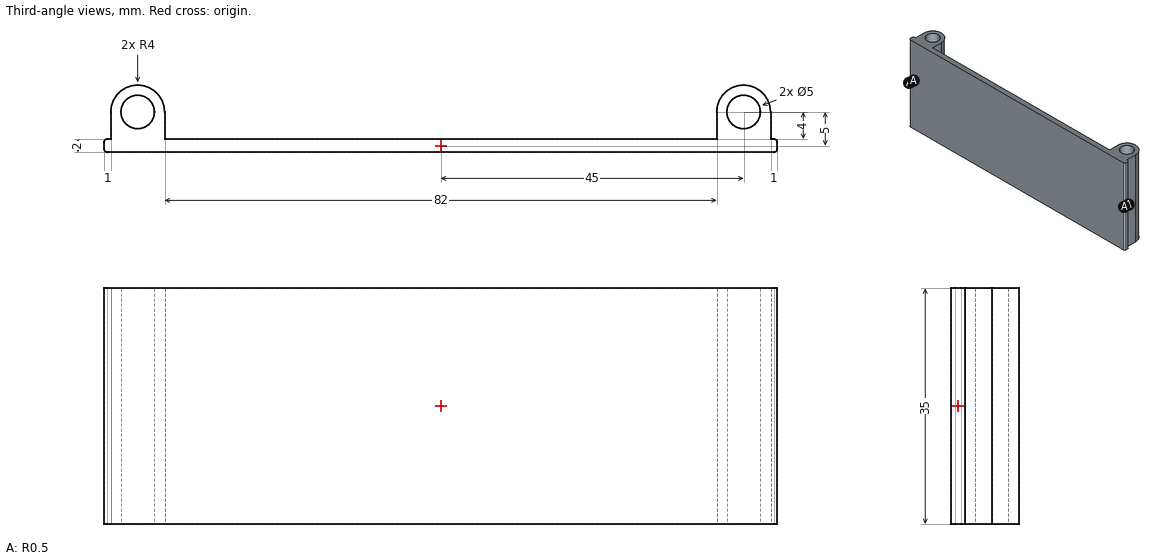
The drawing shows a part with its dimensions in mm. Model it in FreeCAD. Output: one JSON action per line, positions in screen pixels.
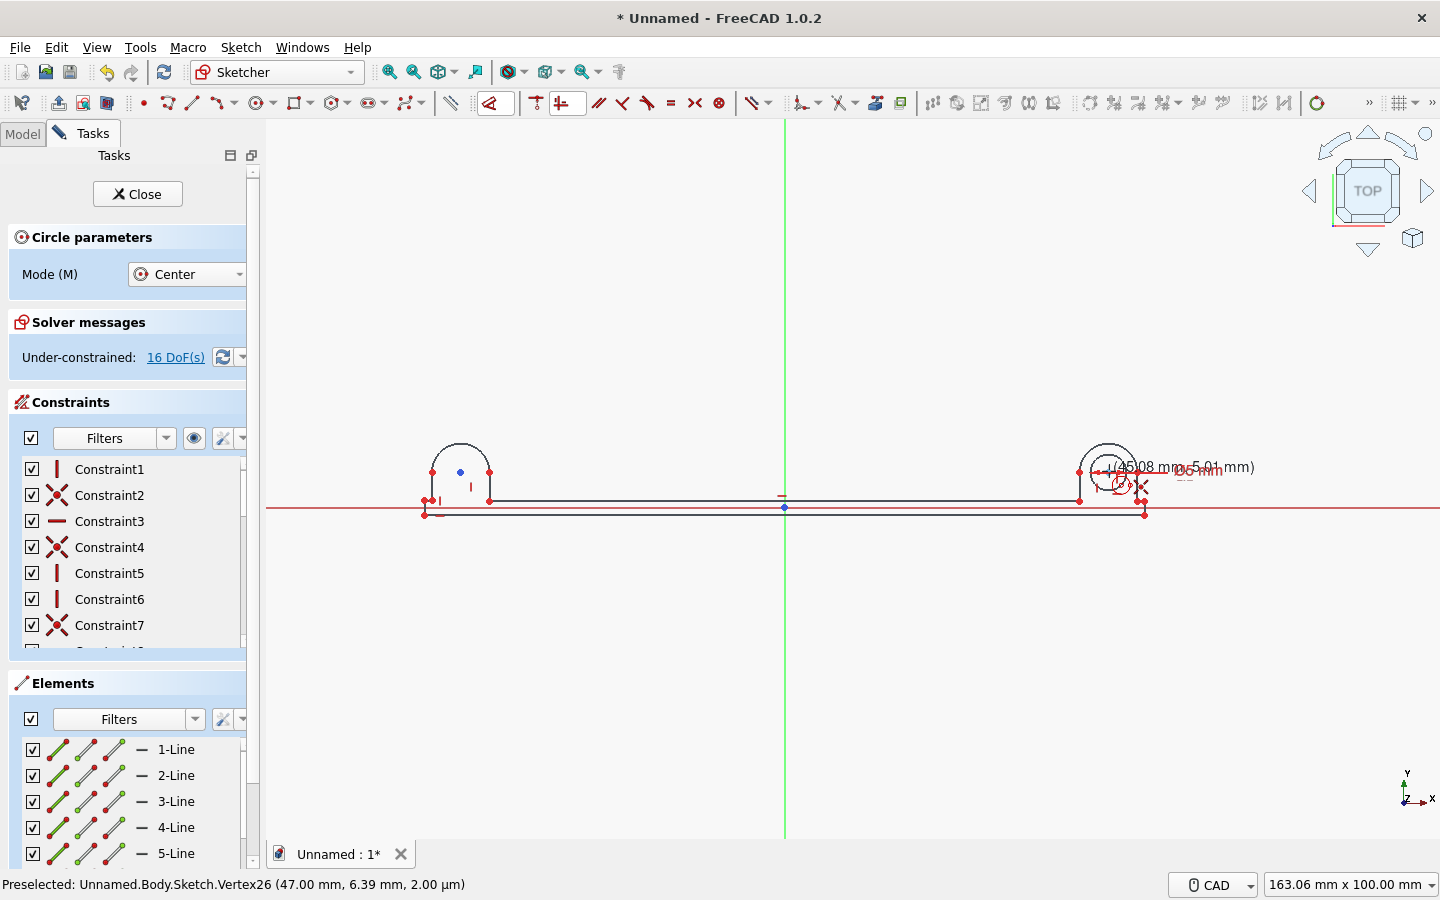
{"action": "scroll", "coordinate": [461, 472], "scroll_direction": "up", "scroll_amount": 2}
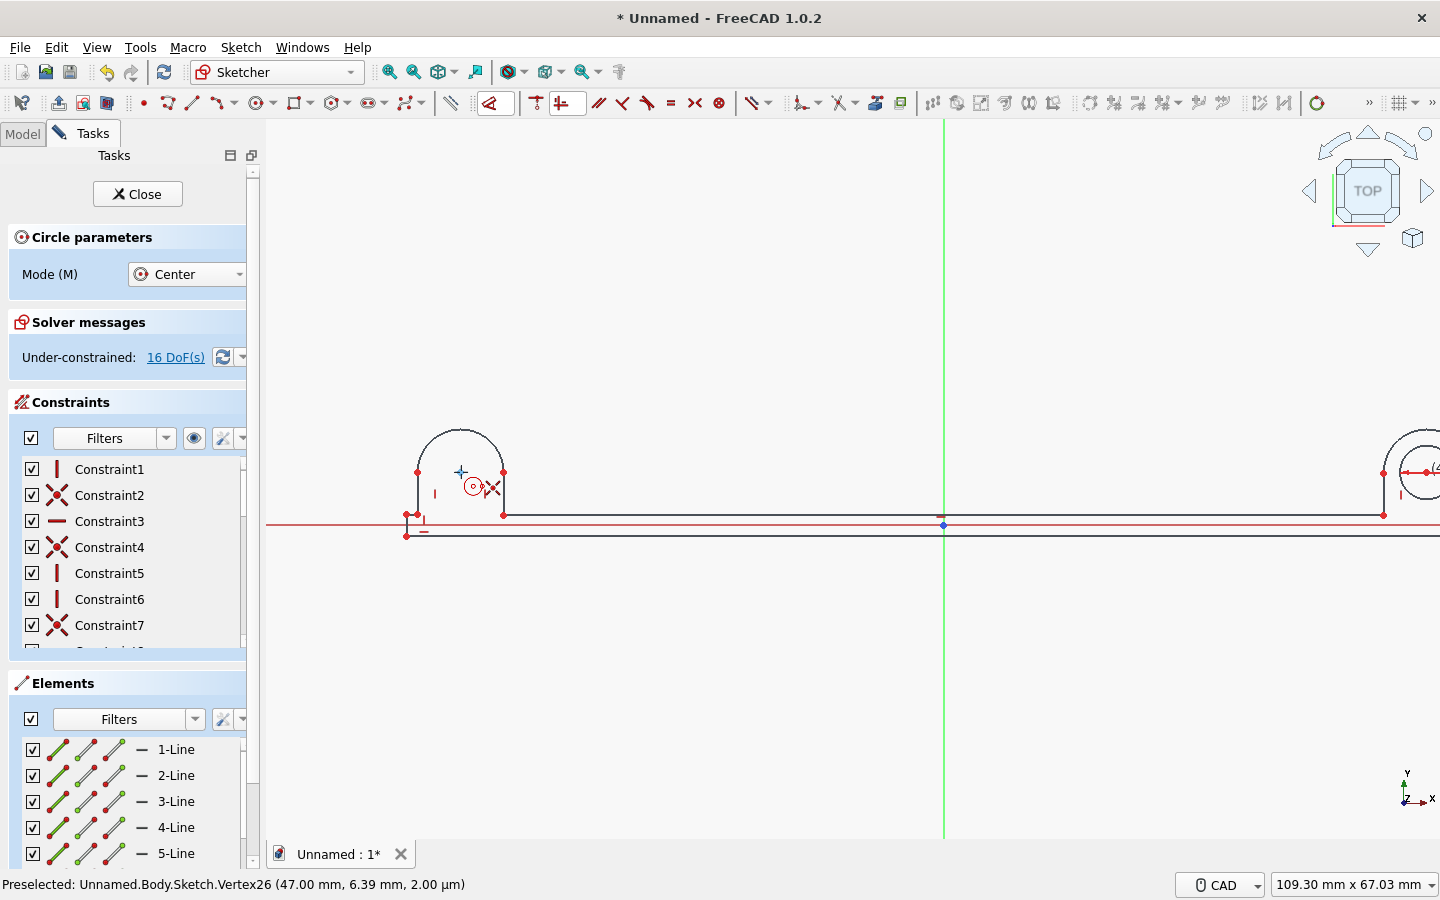
{"action": "left_click", "coordinate": [460, 472]}
{"action": "mouse_move", "coordinate": [479, 453]}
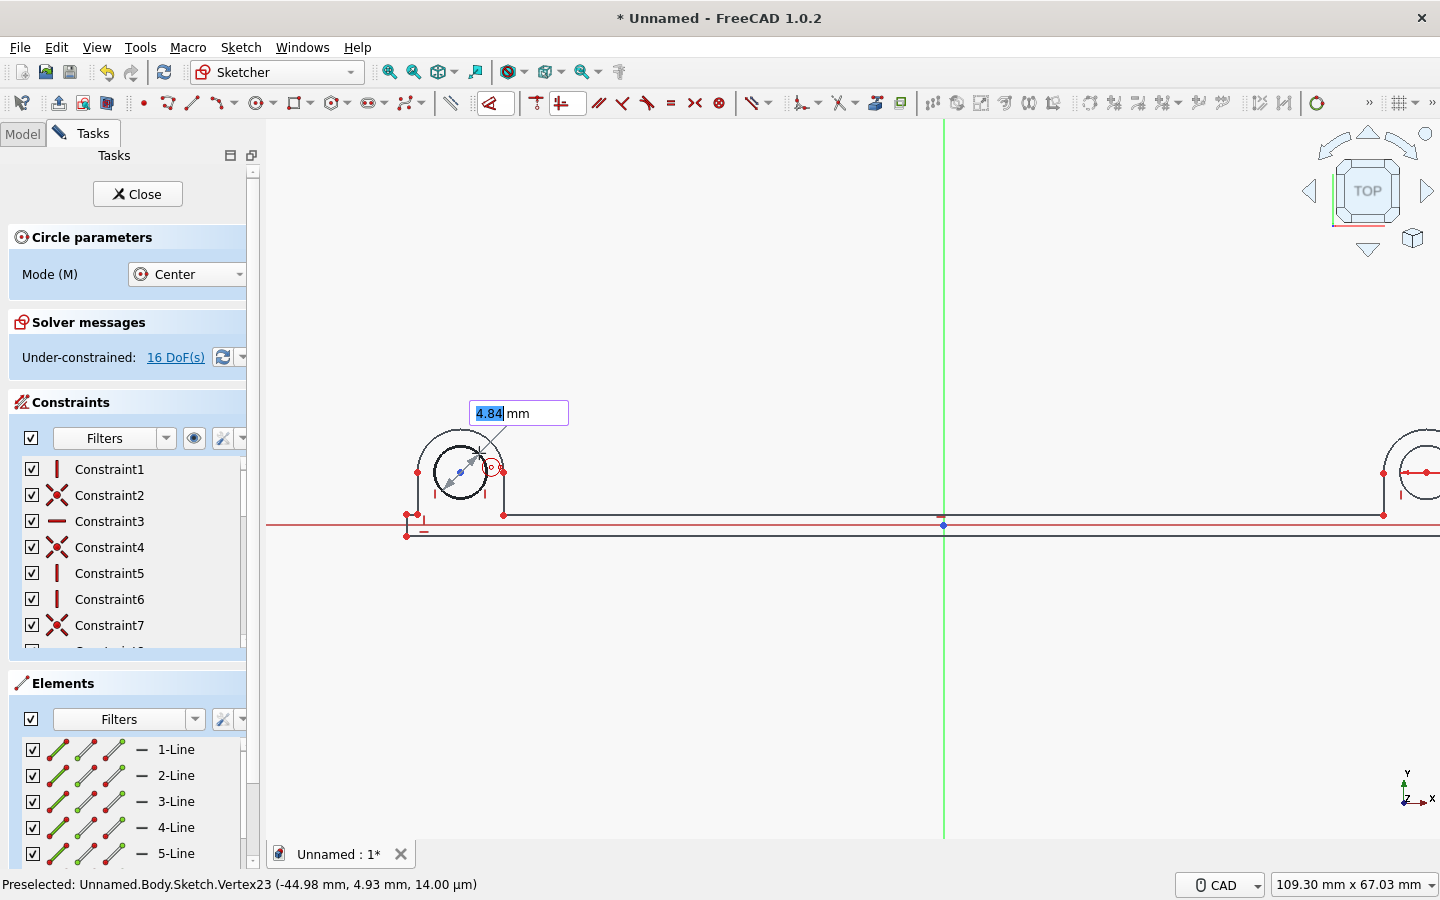
{"action": "type", "text": "5"}
{"action": "key", "text": "Return"}
{"action": "key", "text": "Escape"}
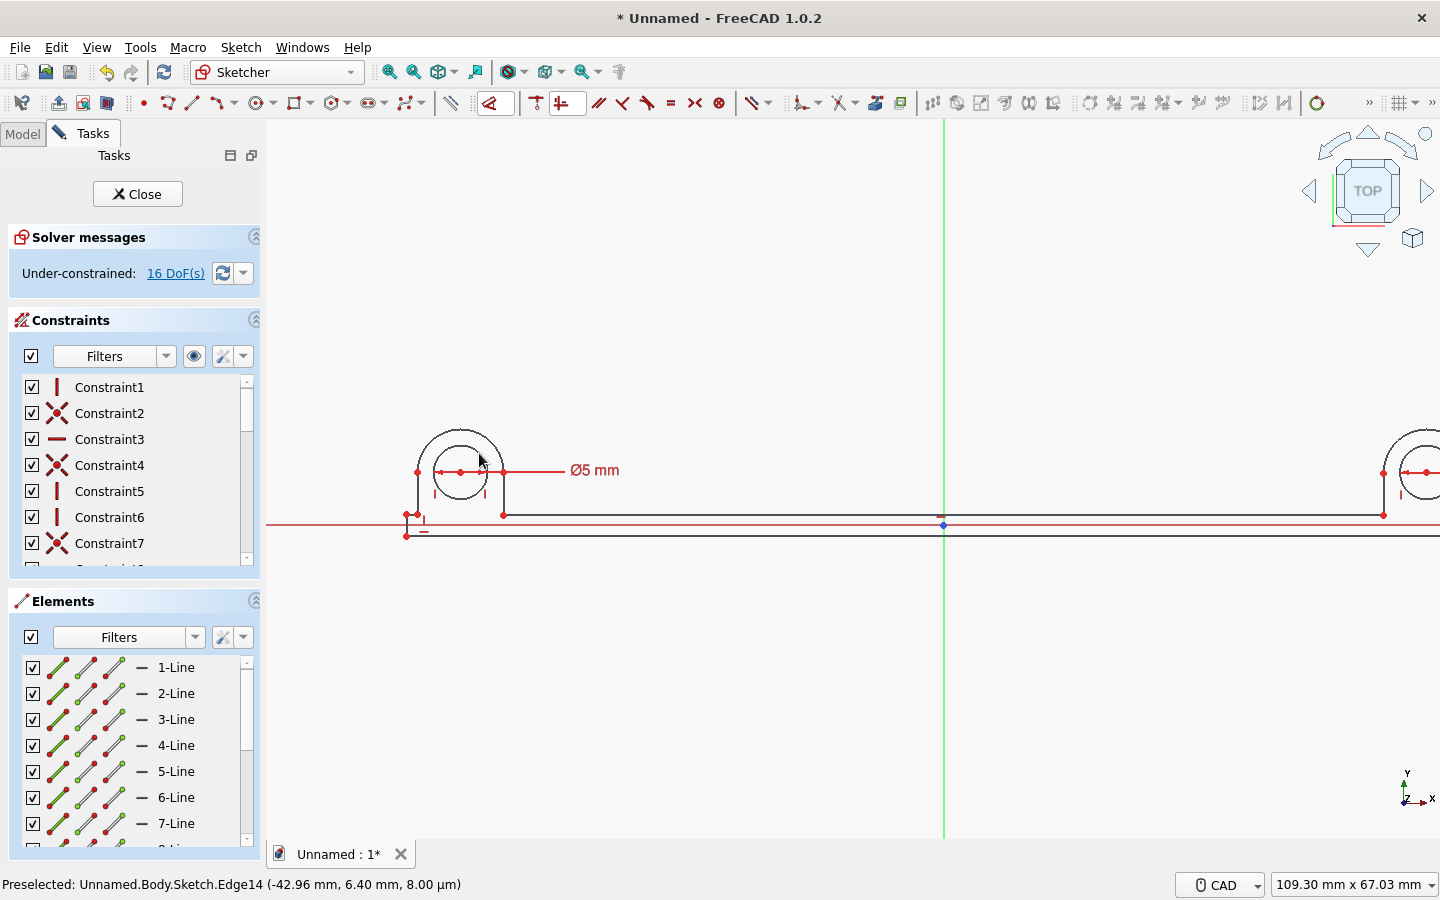
{"action": "scroll", "coordinate": [461, 472], "scroll_direction": "down", "scroll_amount": 2}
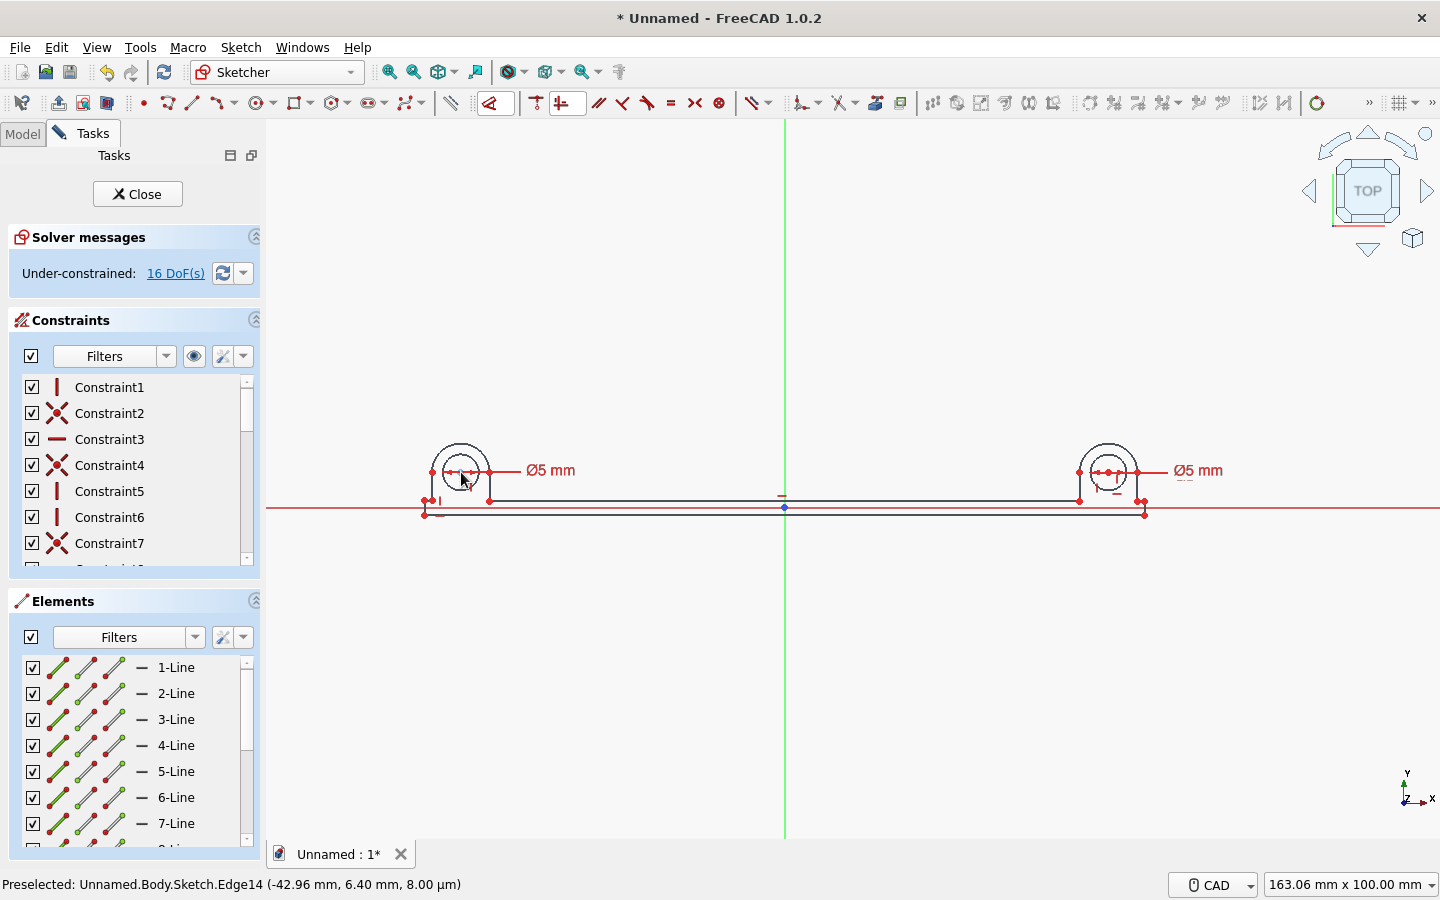
{"action": "scroll", "coordinate": [1080, 481], "scroll_direction": "up", "scroll_amount": 3}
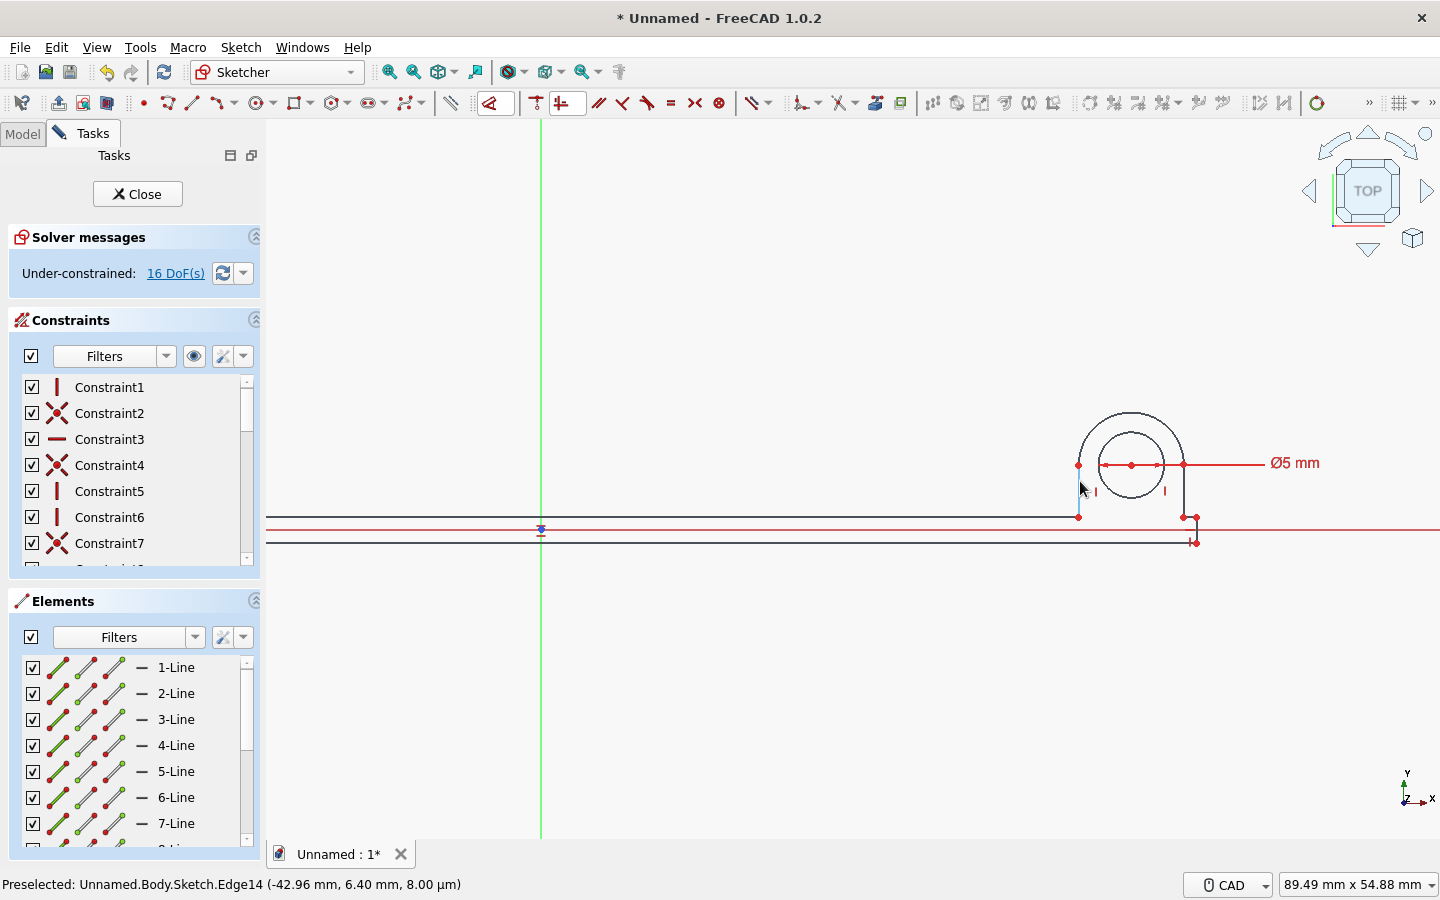
{"action": "left_click", "coordinate": [1079, 481]}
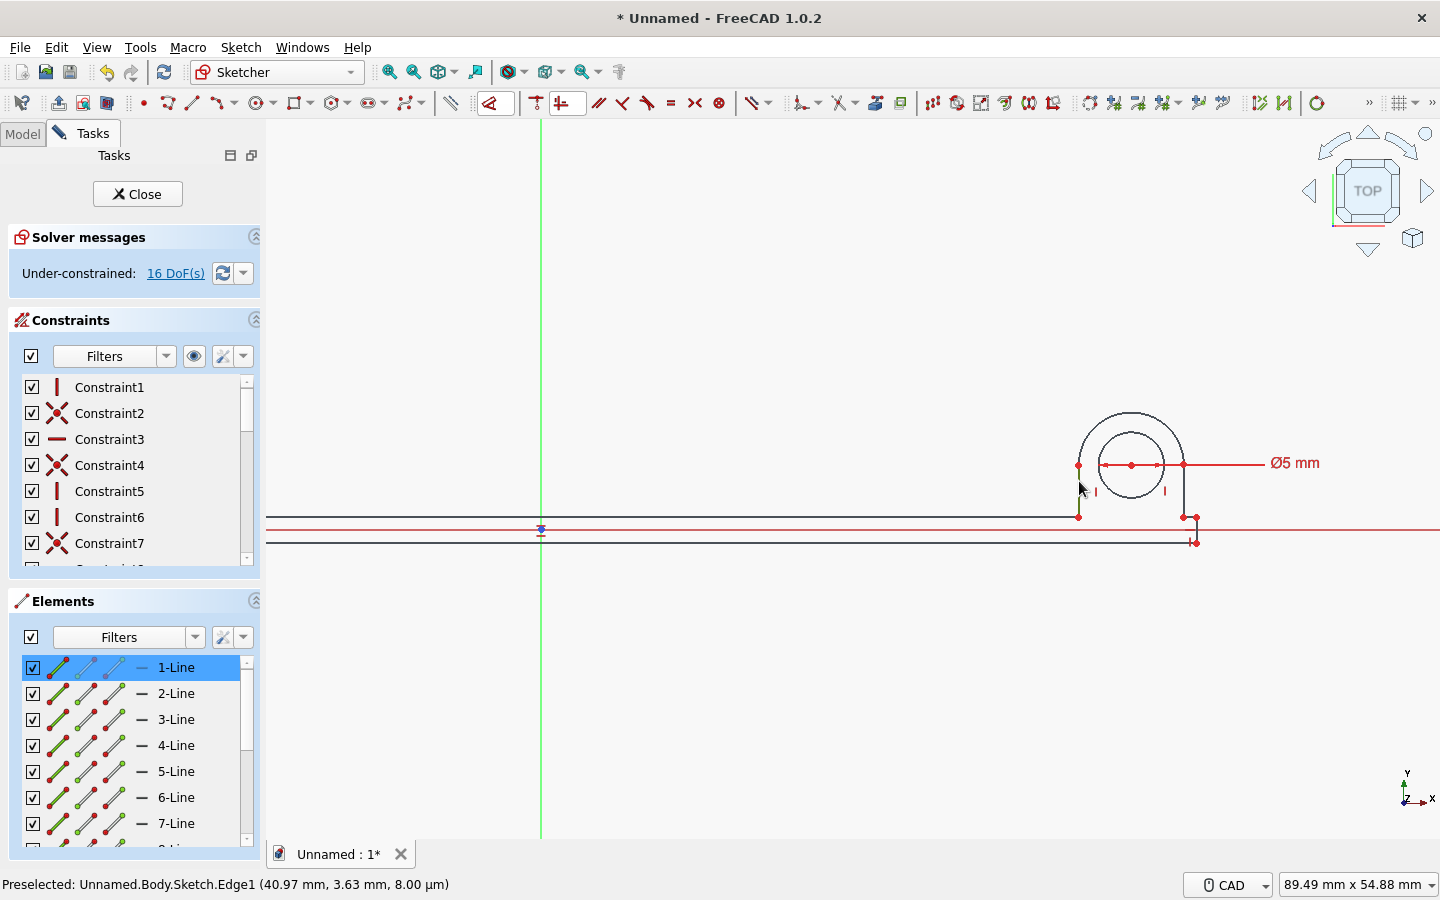
{"action": "left_click", "coordinate": [1162, 422]}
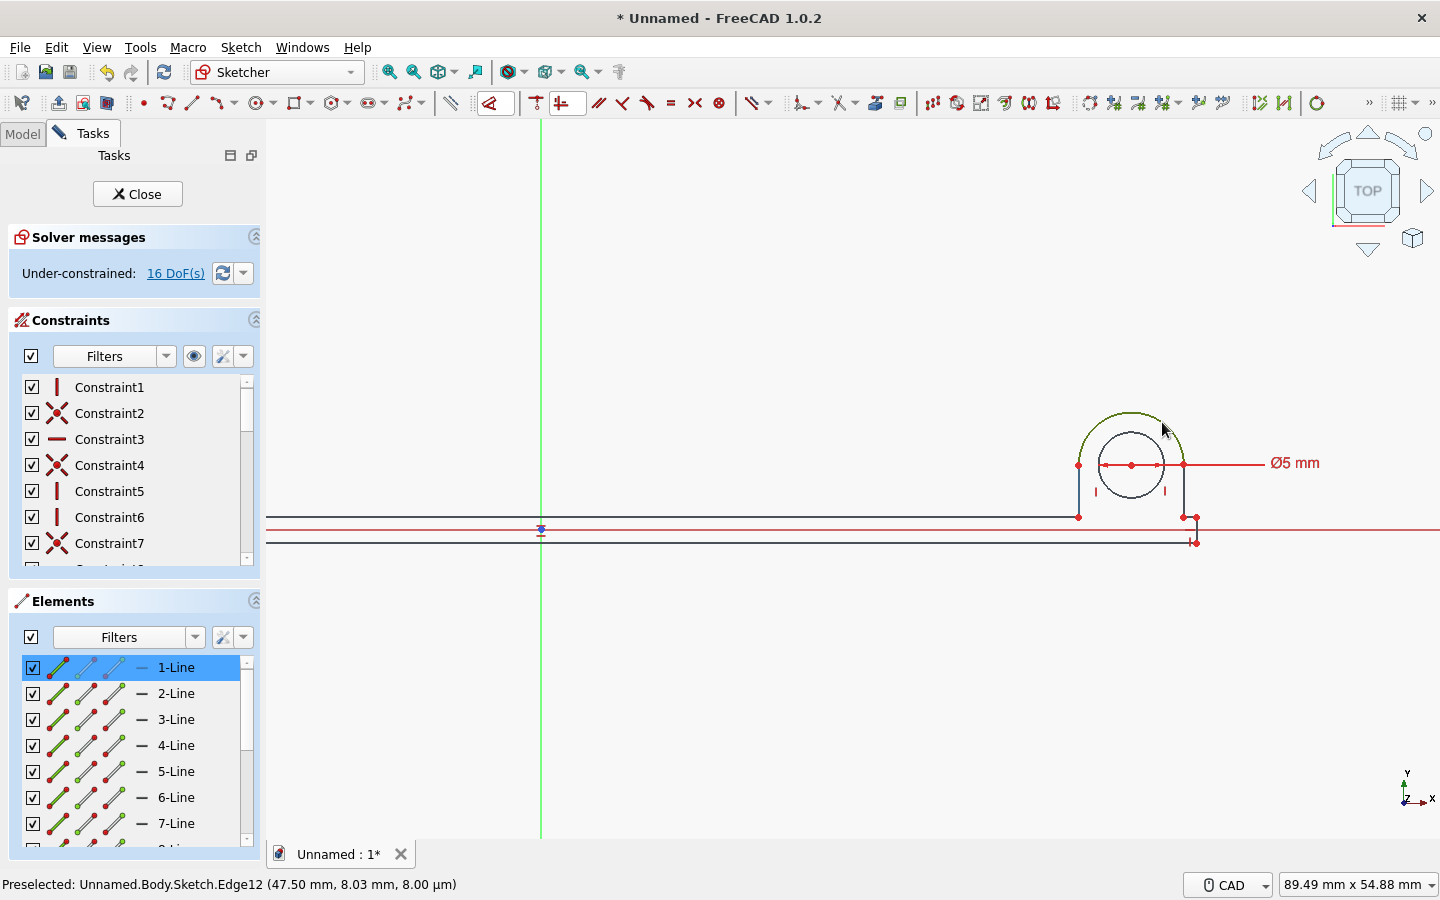
{"action": "left_click", "coordinate": [648, 104]}